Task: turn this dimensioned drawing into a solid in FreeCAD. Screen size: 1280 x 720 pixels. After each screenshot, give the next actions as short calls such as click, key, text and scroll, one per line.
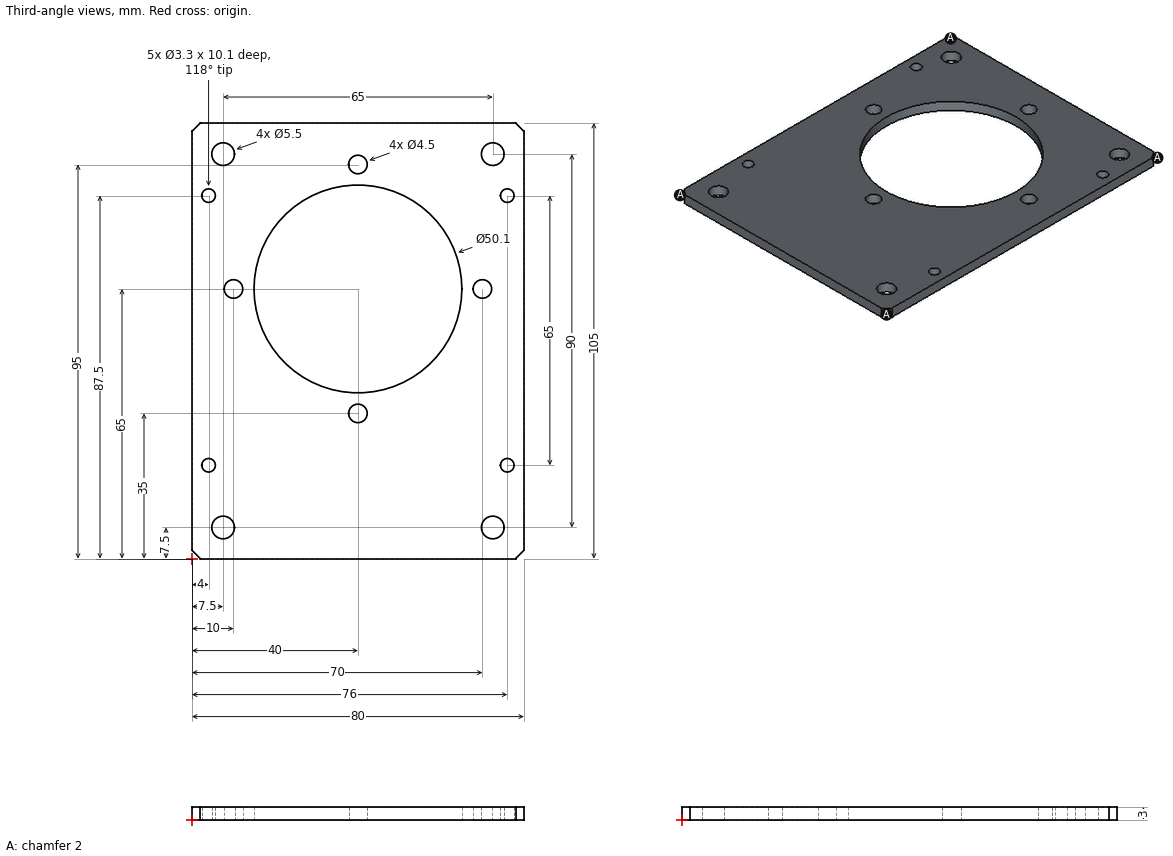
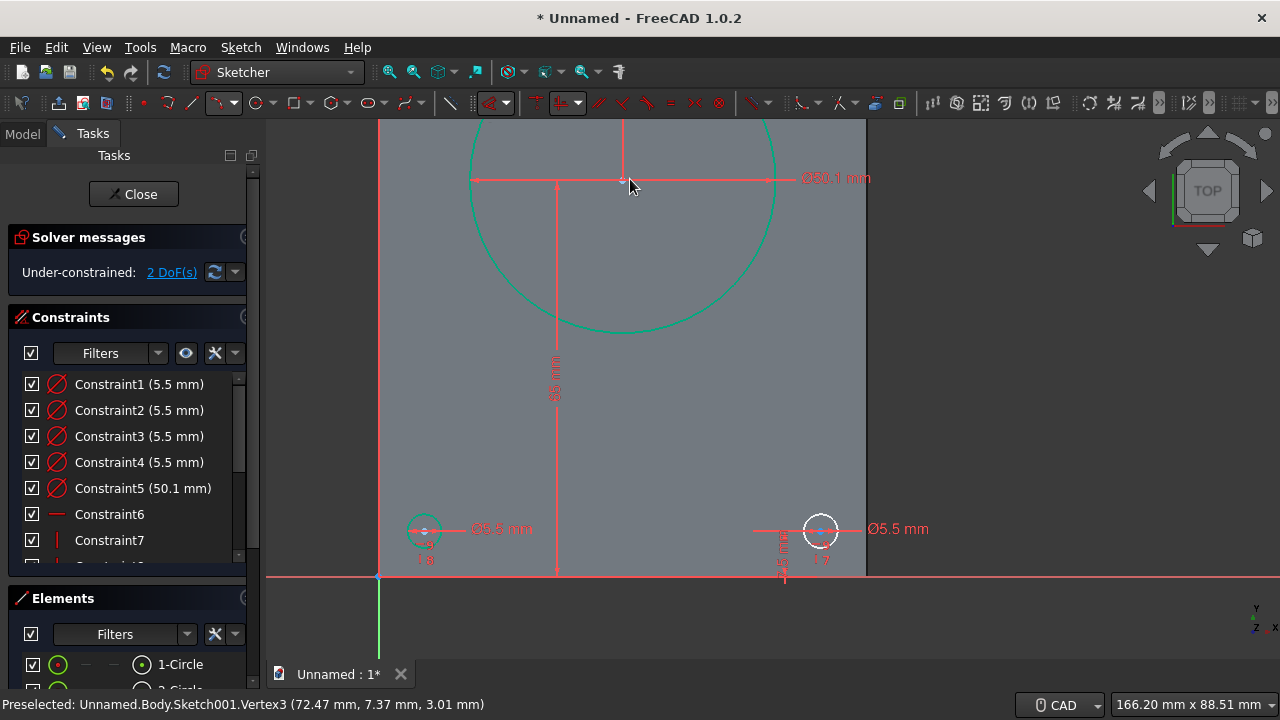
scroll(822, 532, down, 3)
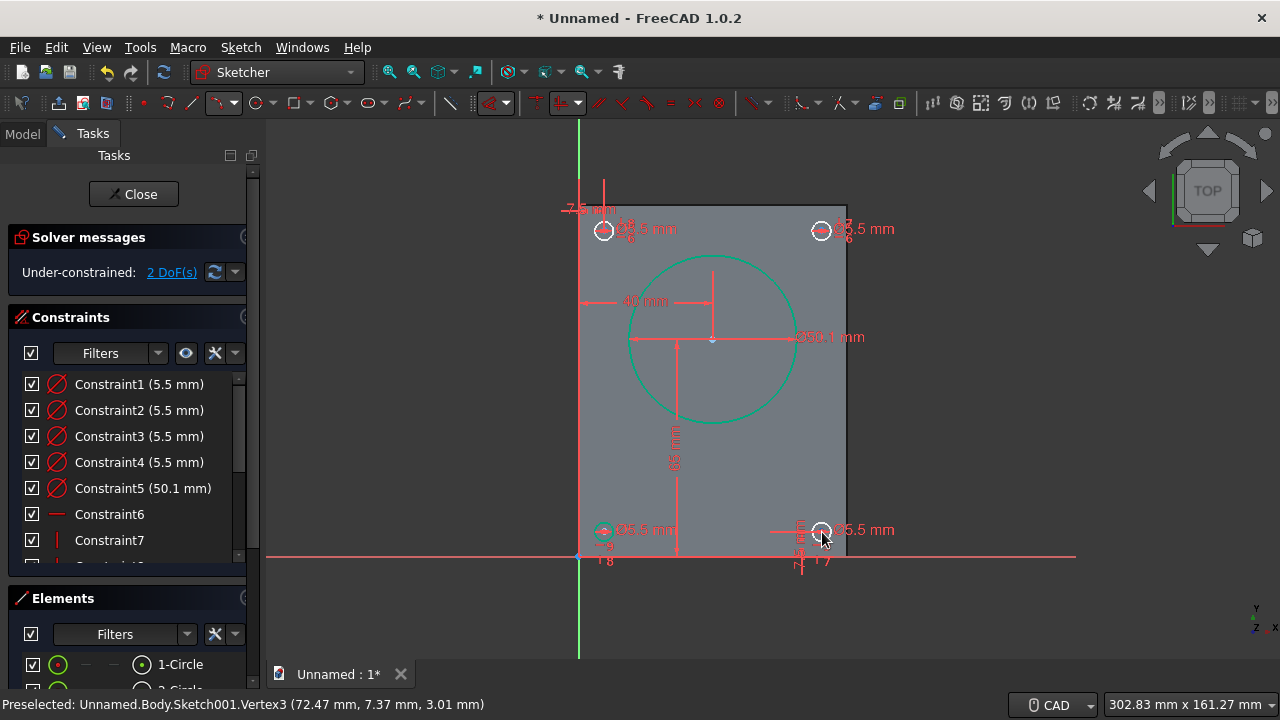
click(604, 231)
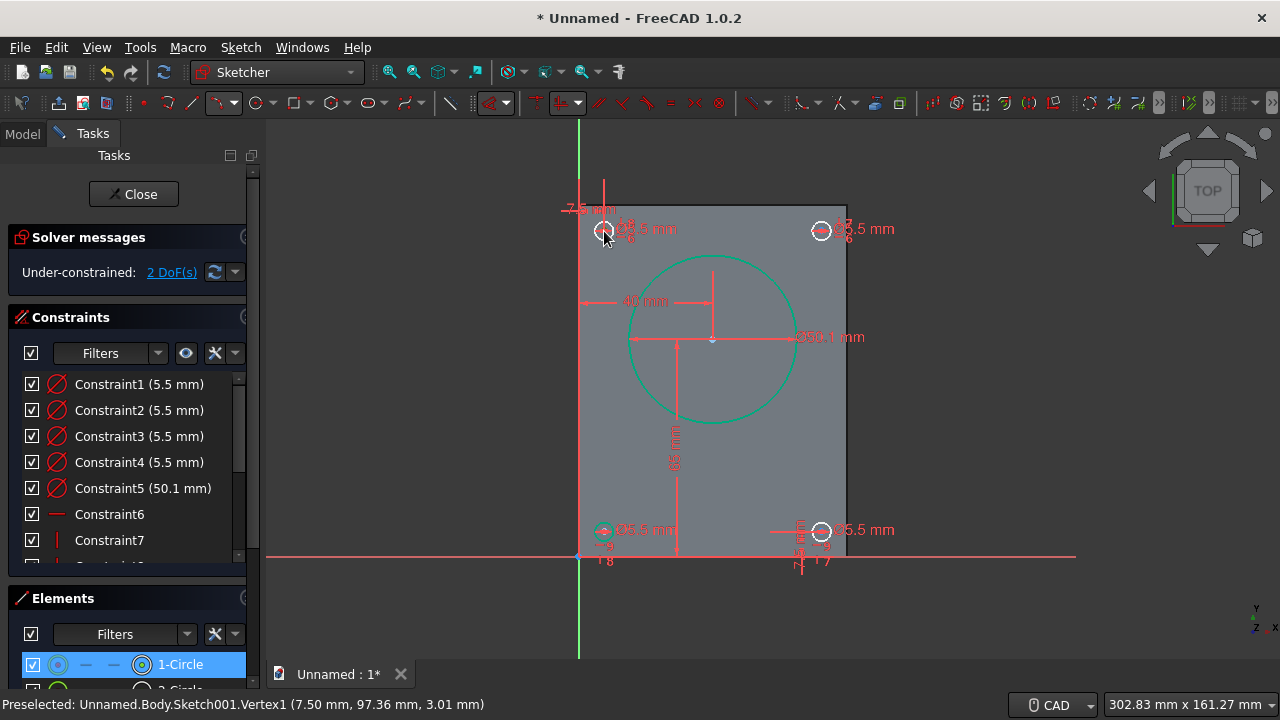
click(822, 231)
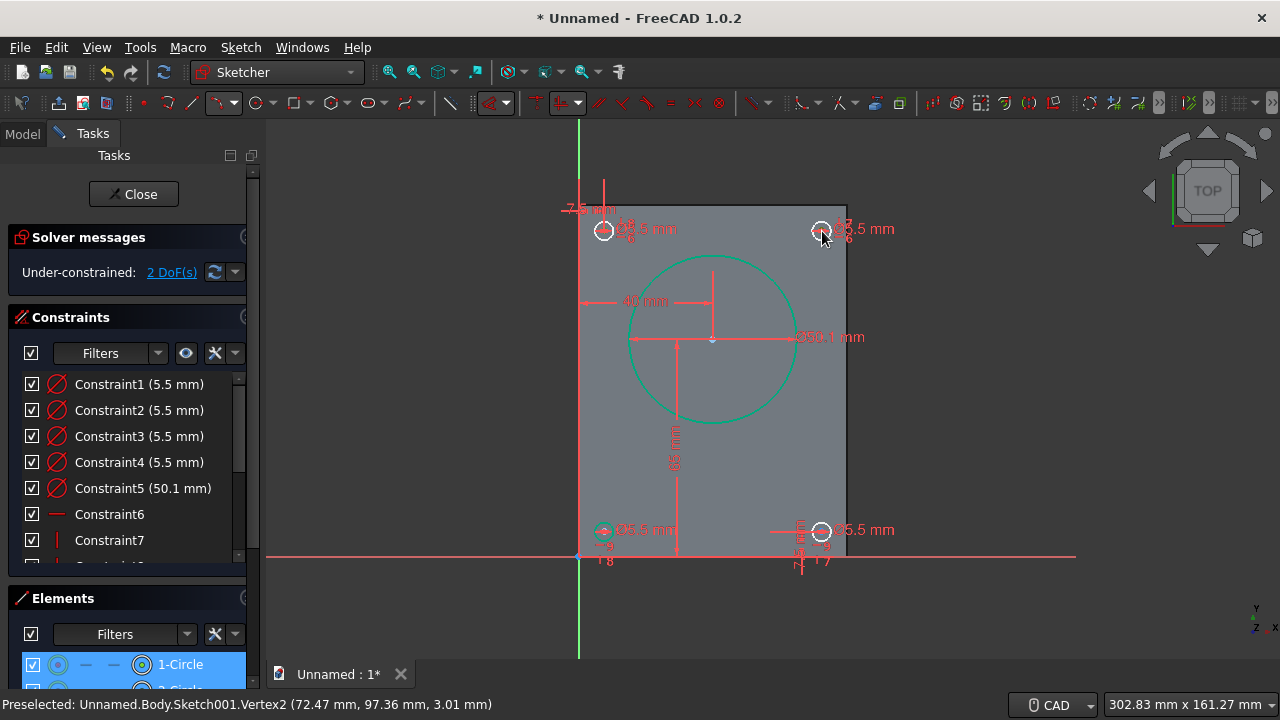
key(l)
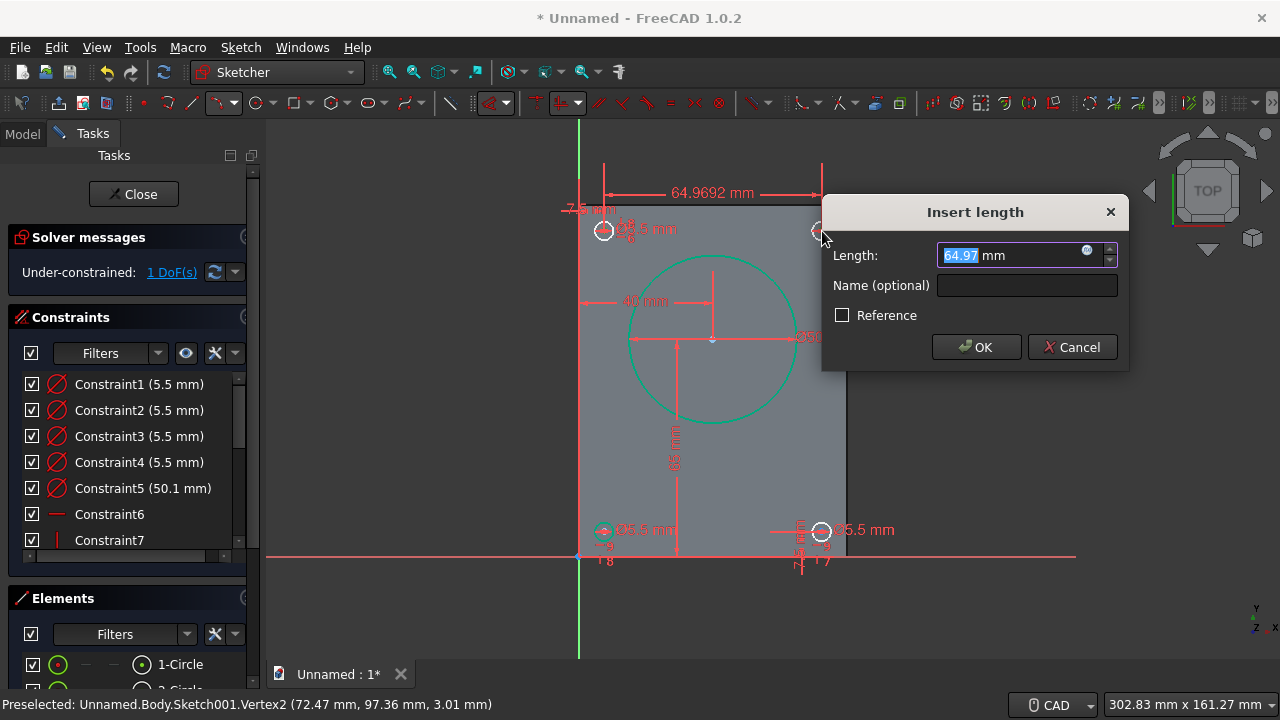
text(65)
key(Return)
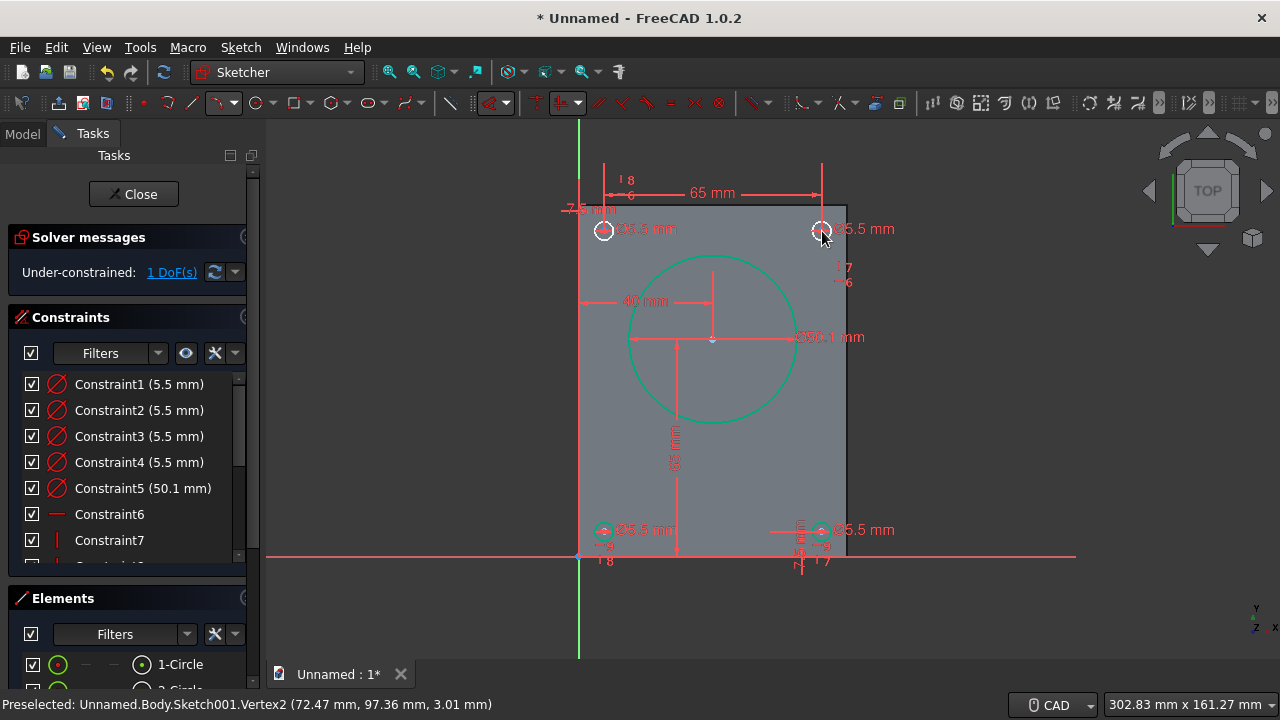
click(822, 231)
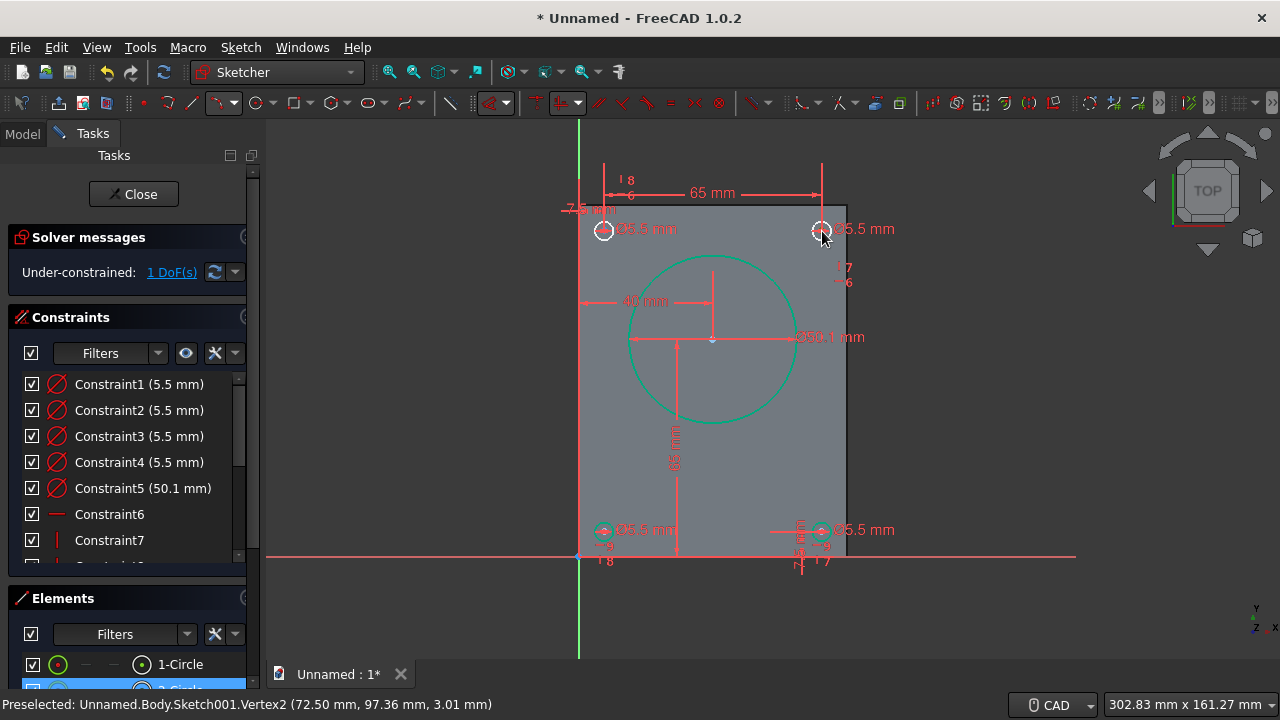
click(822, 532)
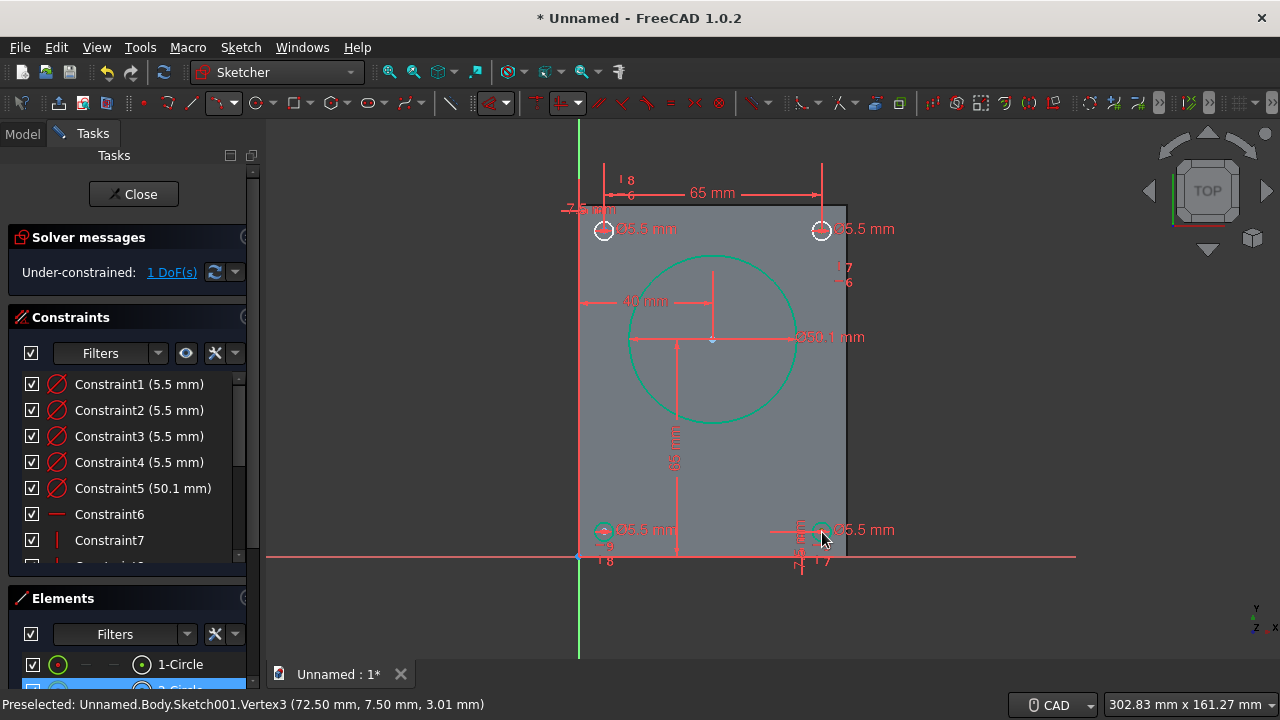
key(i)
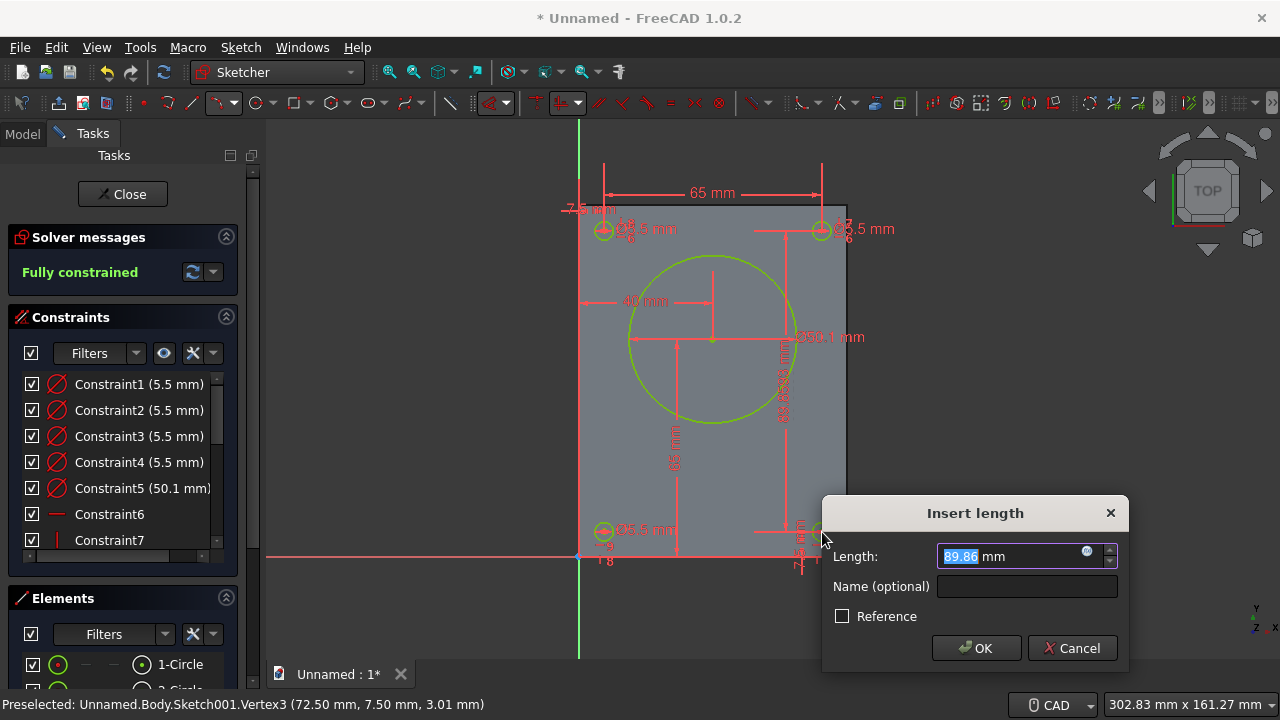
text(90)
key(Return)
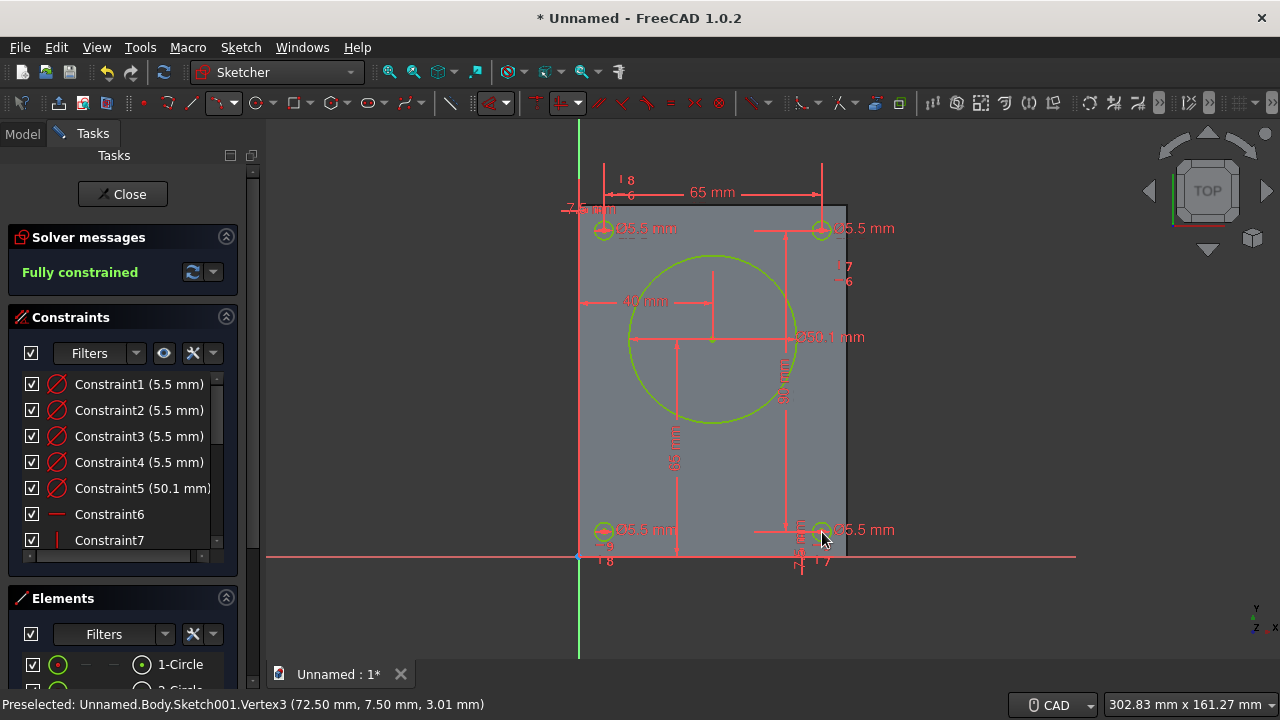
click(123, 194)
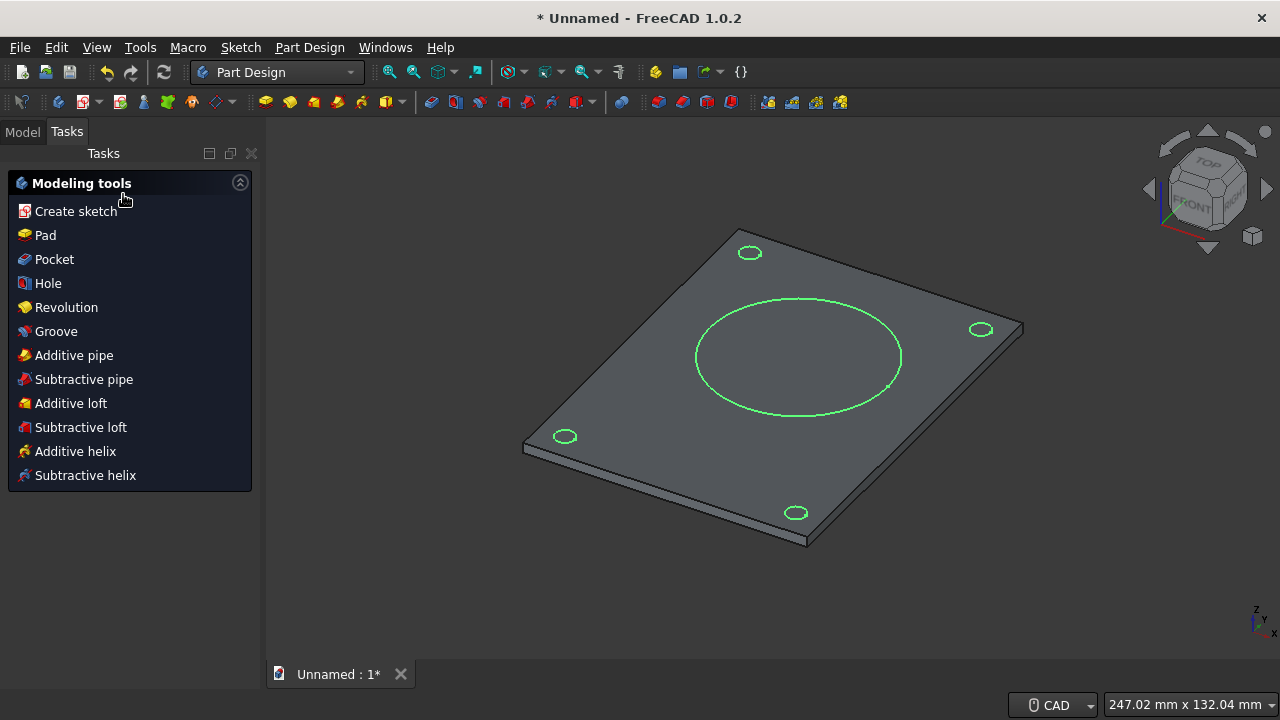
click(432, 102)